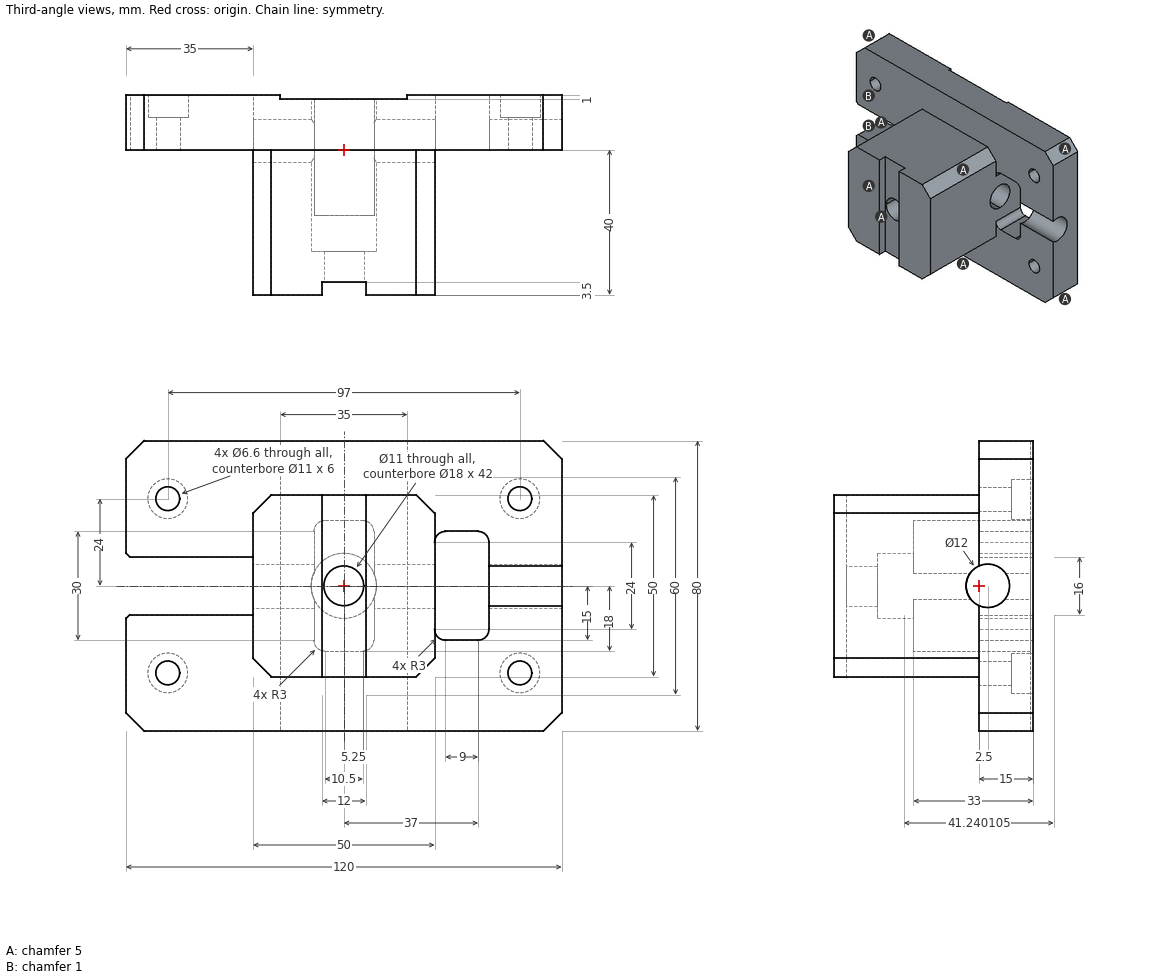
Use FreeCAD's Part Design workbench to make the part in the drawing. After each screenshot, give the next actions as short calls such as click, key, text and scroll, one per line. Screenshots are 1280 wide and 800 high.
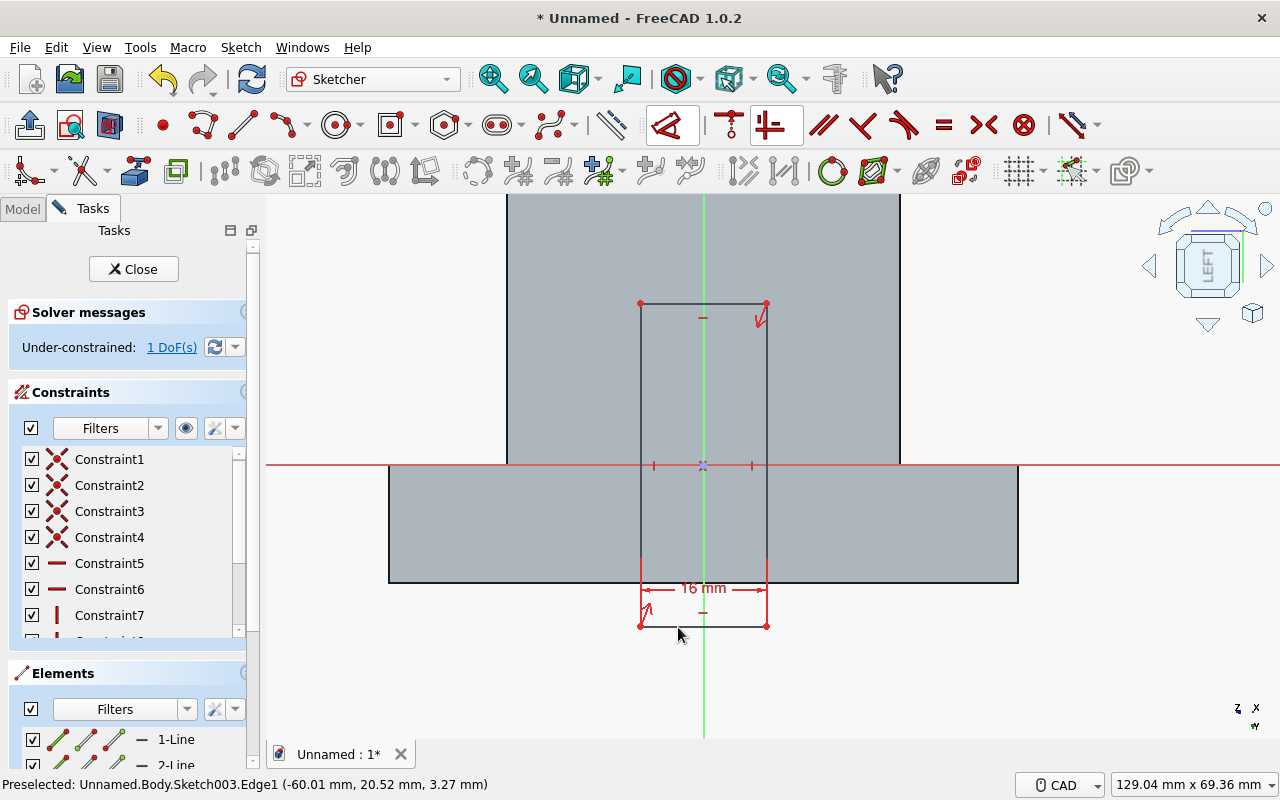
click(767, 530)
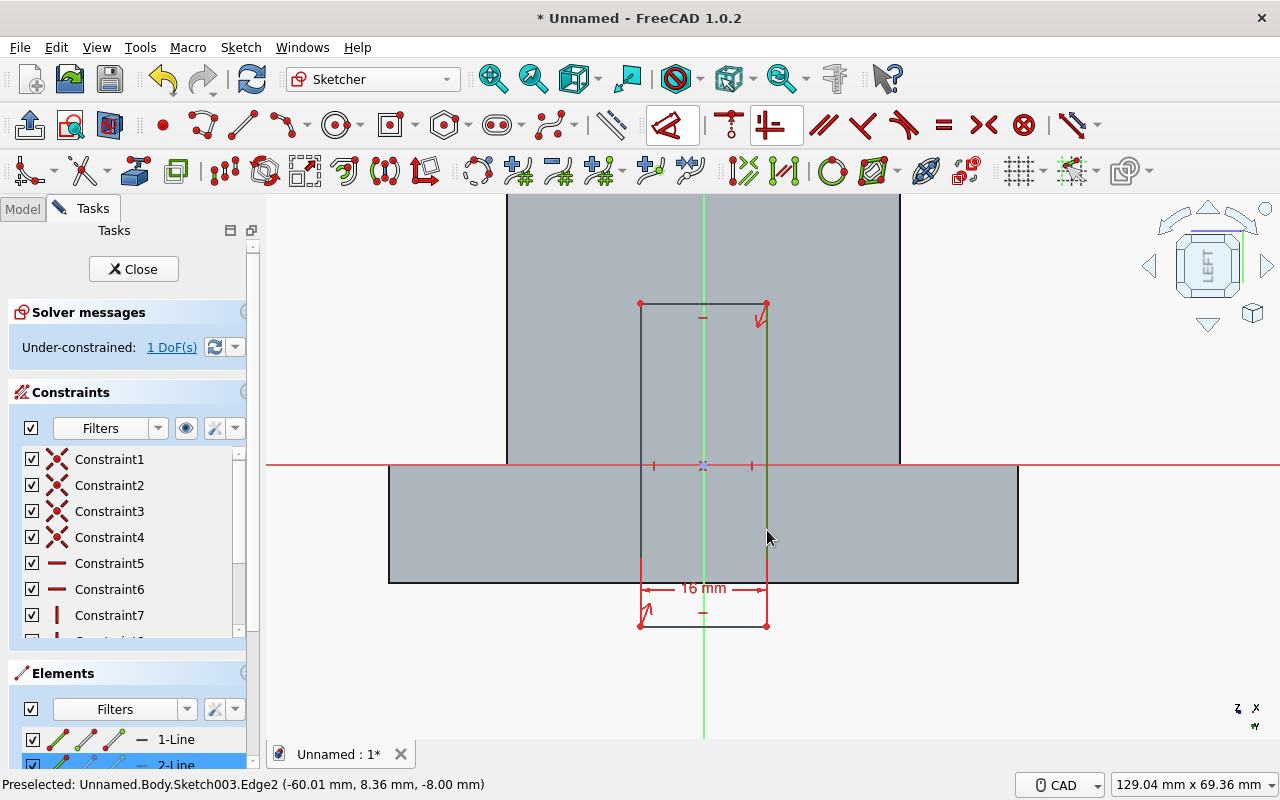
key(i)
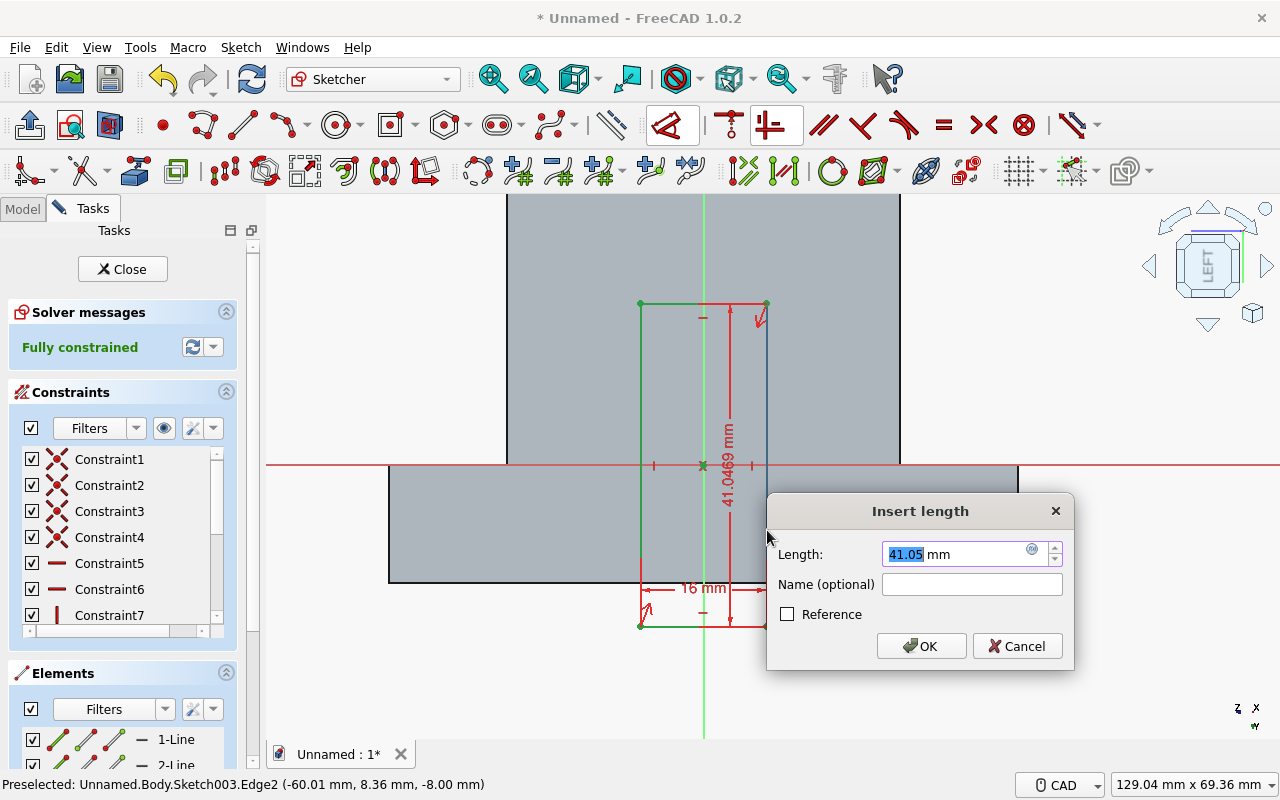
text(41.240105)
key(Return)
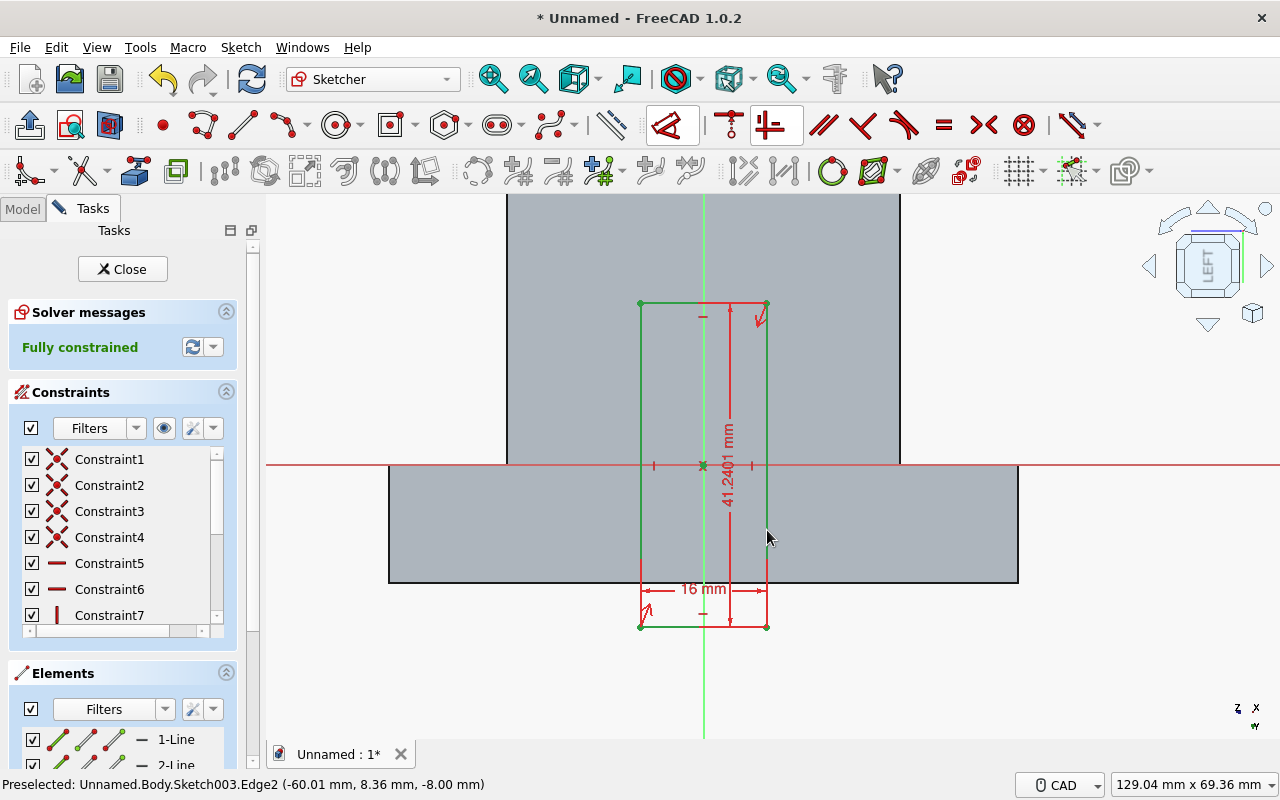
click(123, 269)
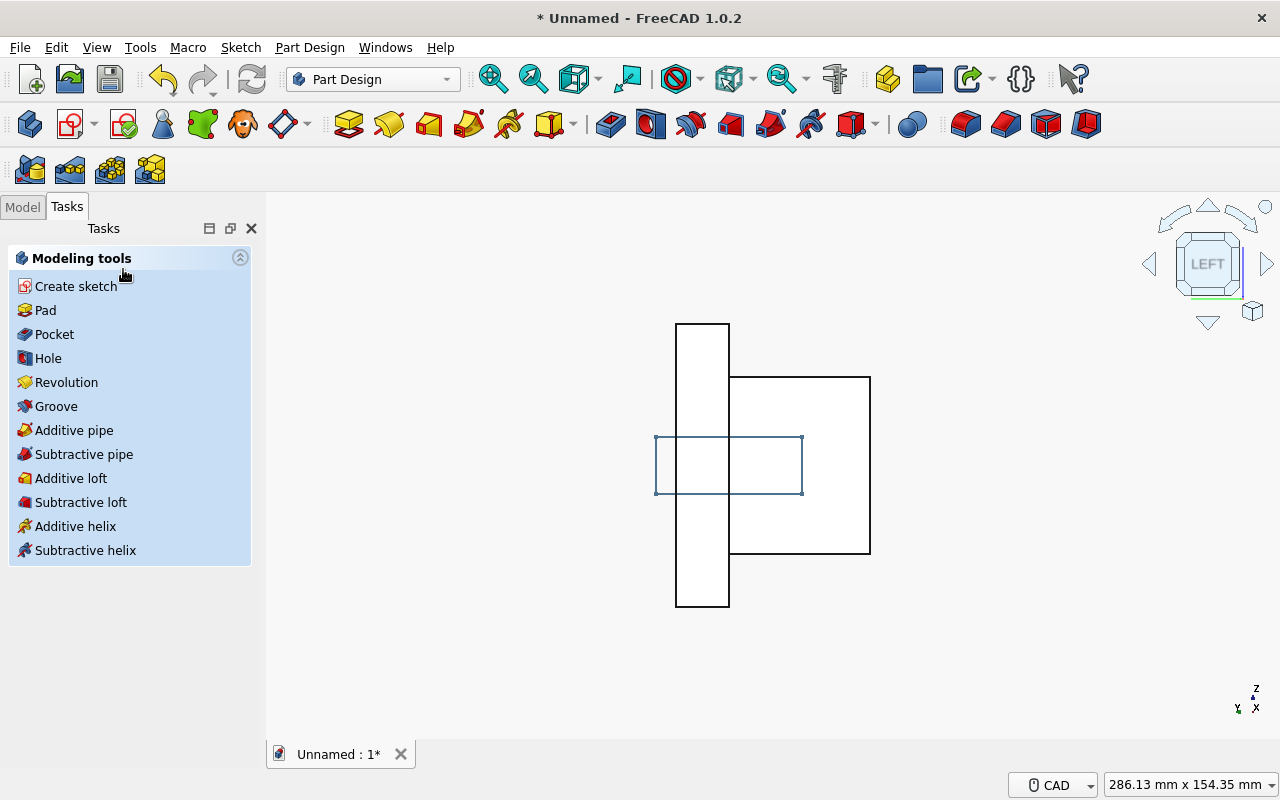
click(612, 124)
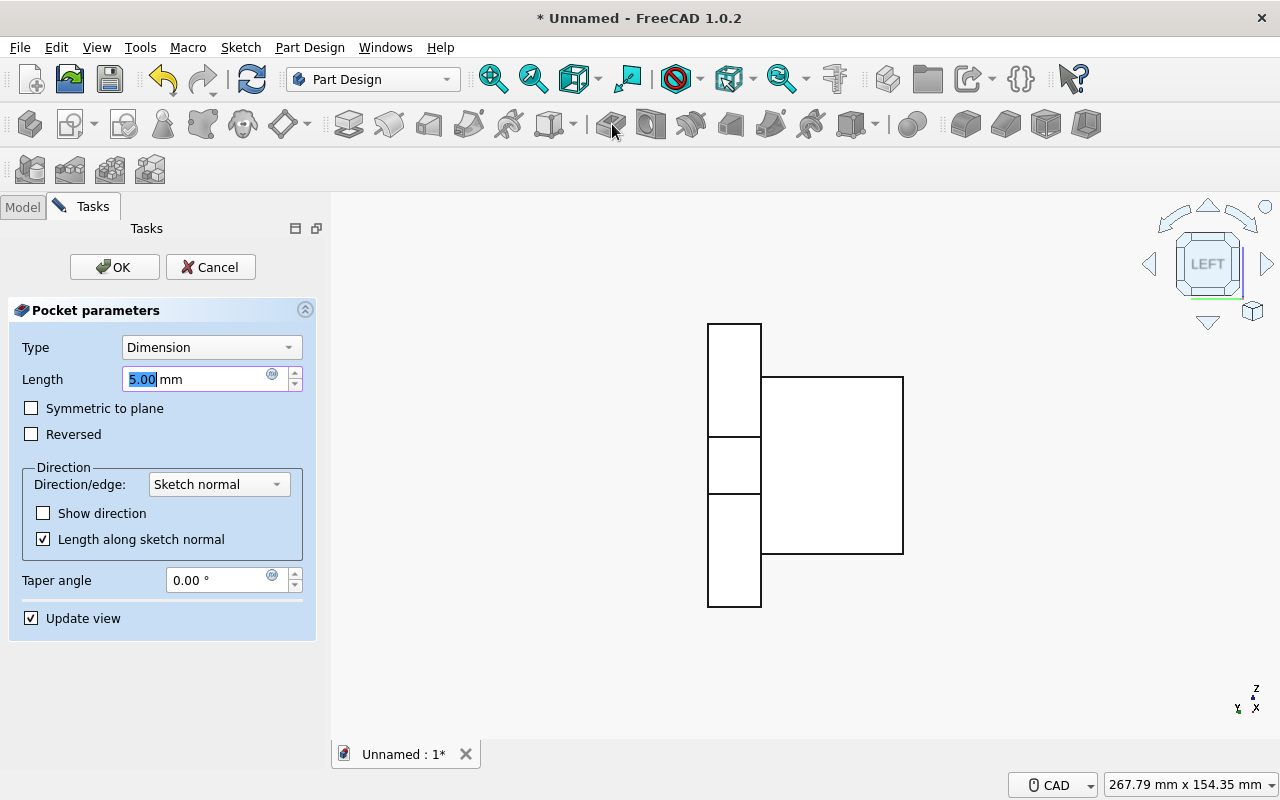
text(35)
key(Tab)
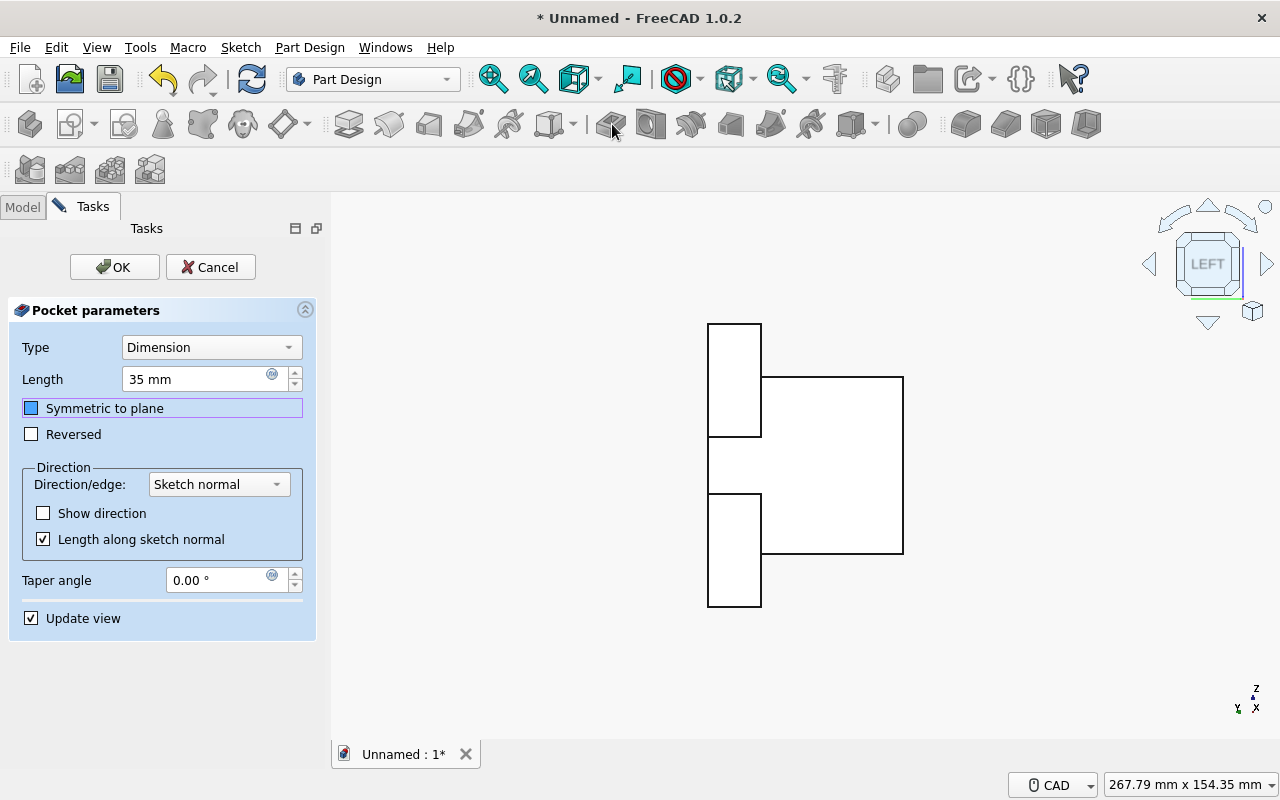
click(115, 267)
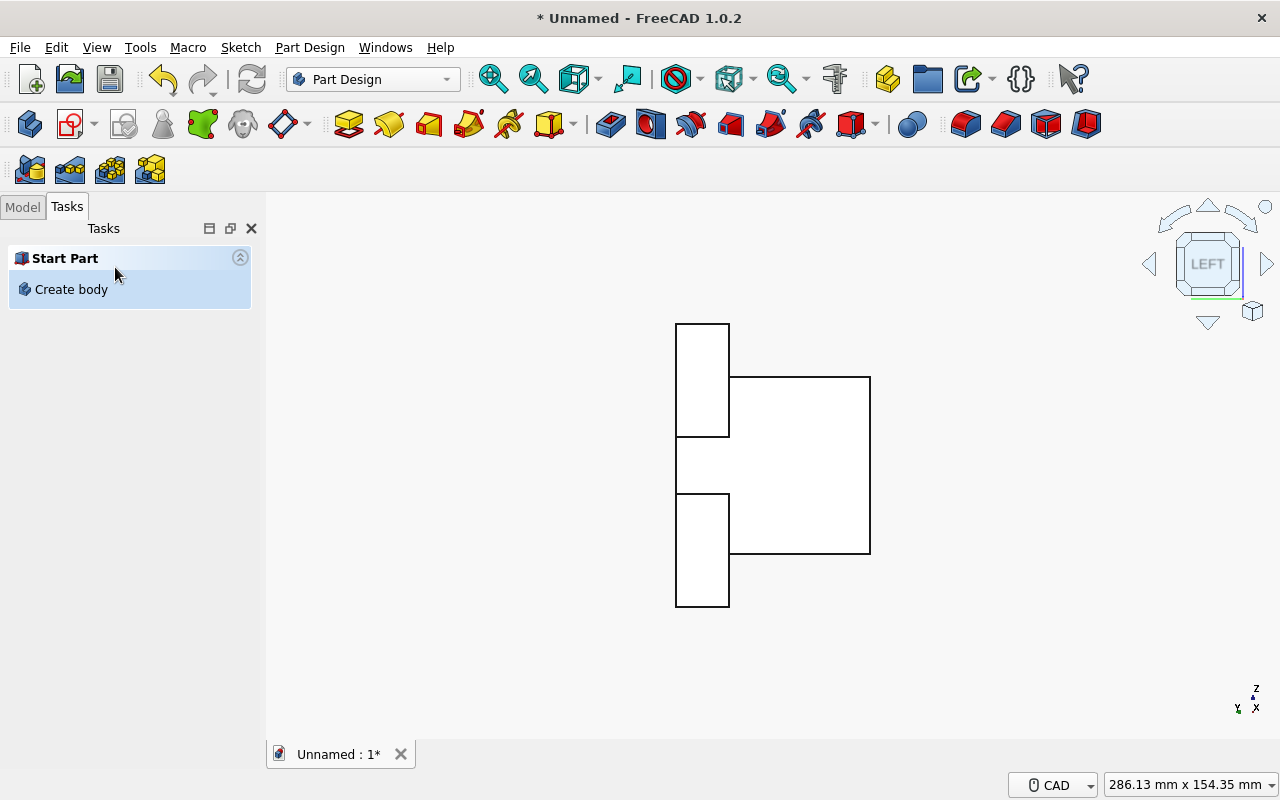
click(801, 465)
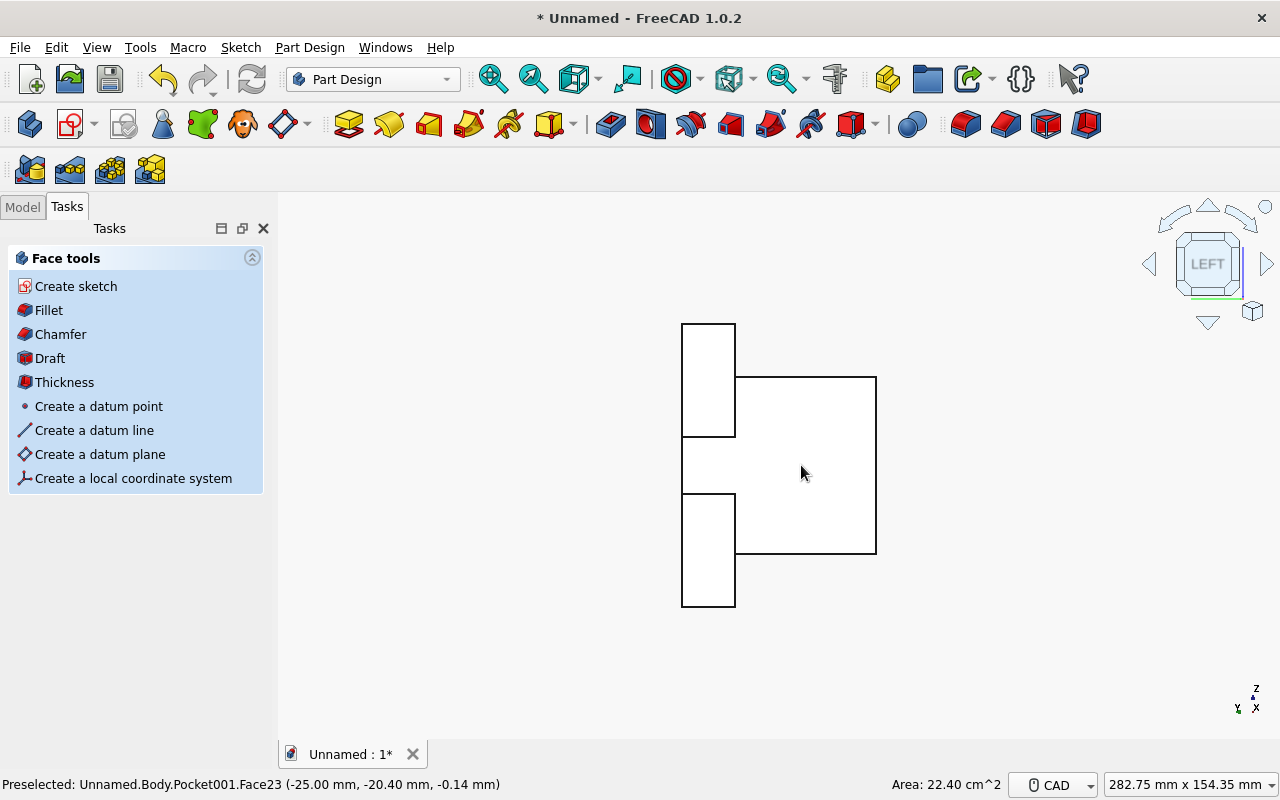
click(70, 124)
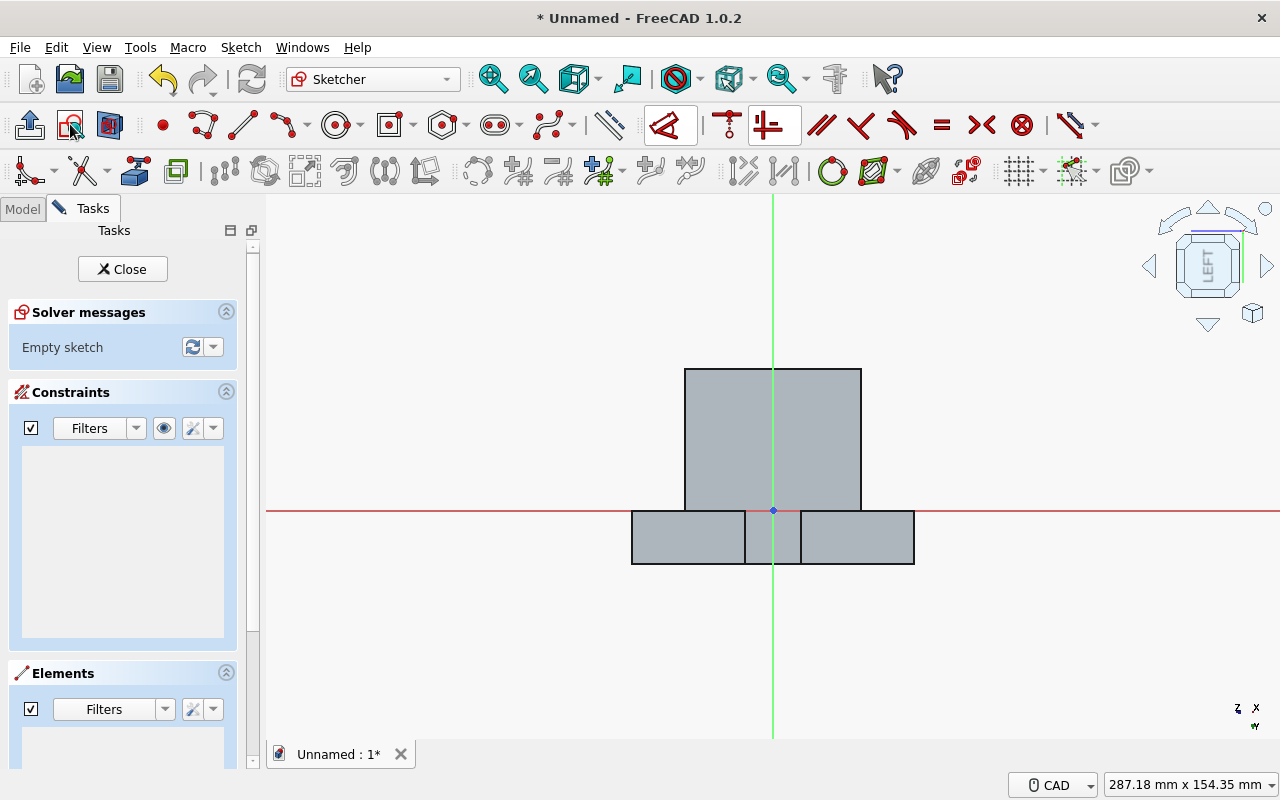
scroll(784, 528, up, 10)